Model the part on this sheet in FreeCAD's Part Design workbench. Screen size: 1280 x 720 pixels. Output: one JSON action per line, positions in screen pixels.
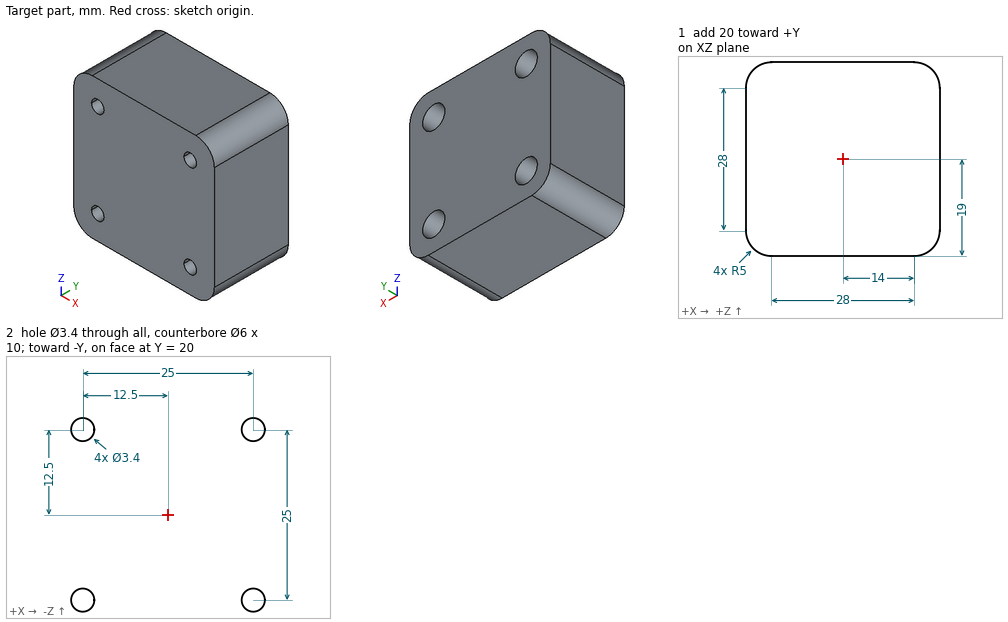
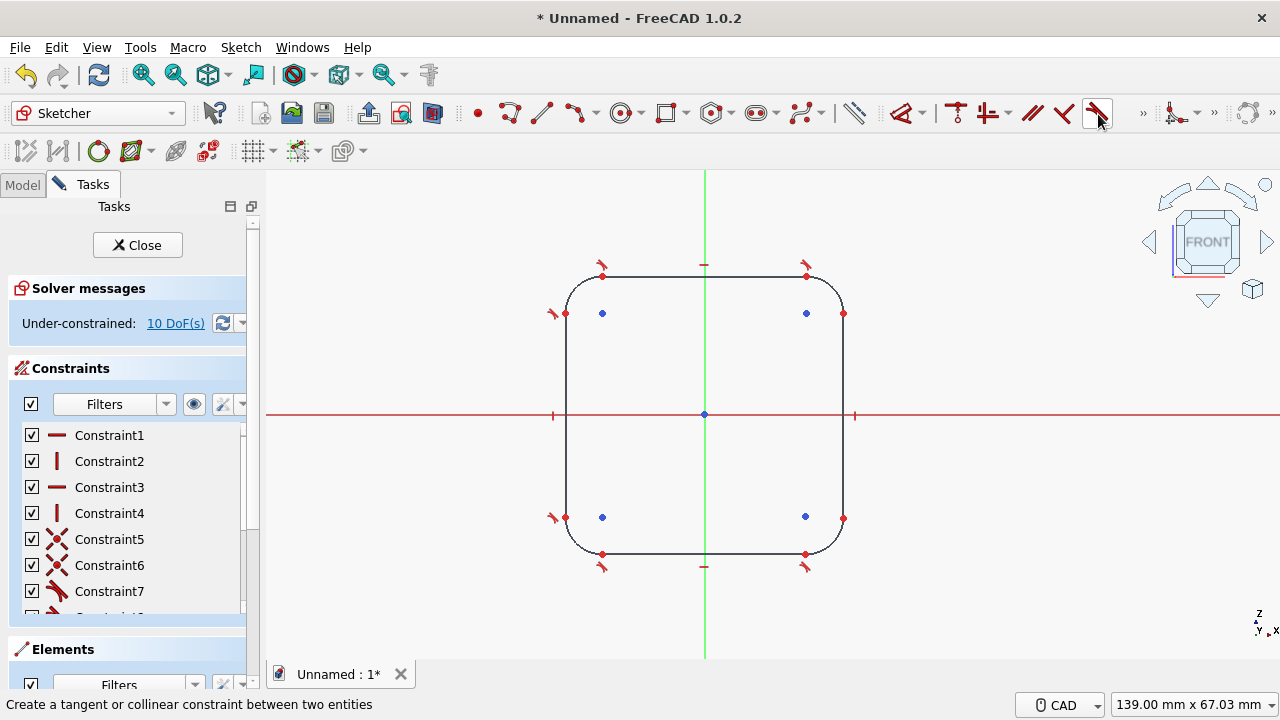
{"action": "left_click", "coordinate": [843, 375]}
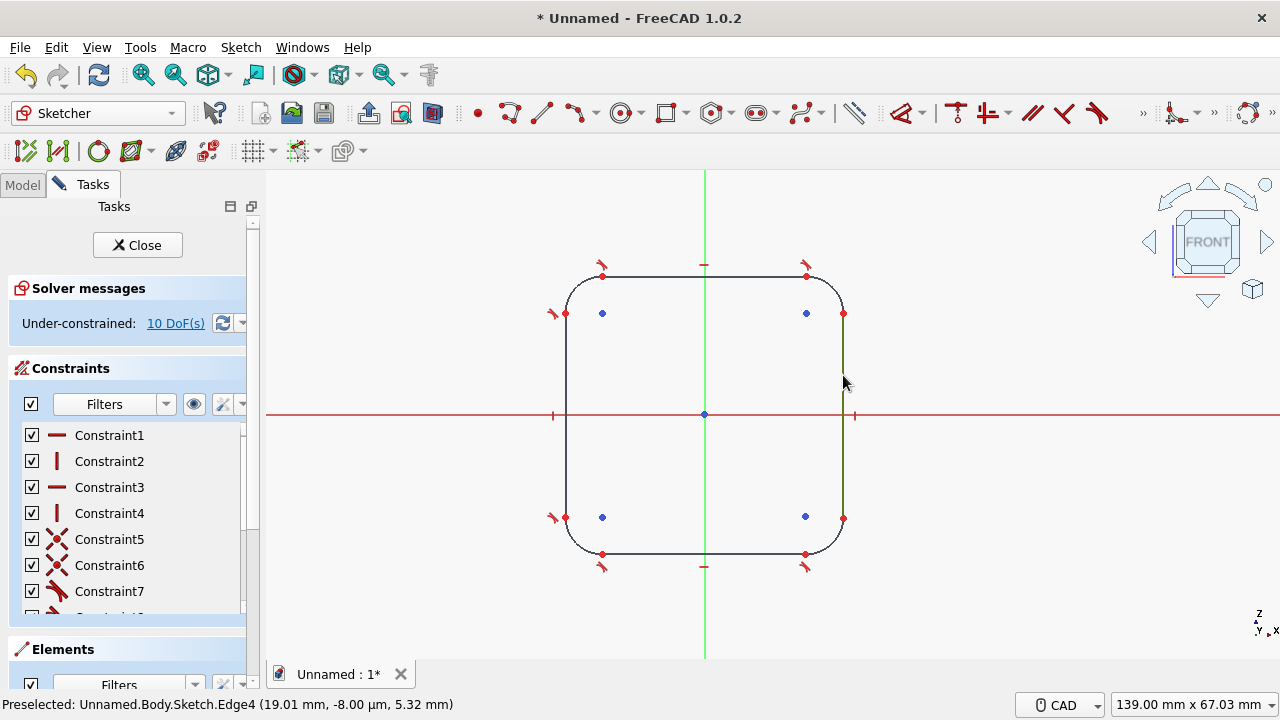
{"action": "left_click", "coordinate": [839, 297]}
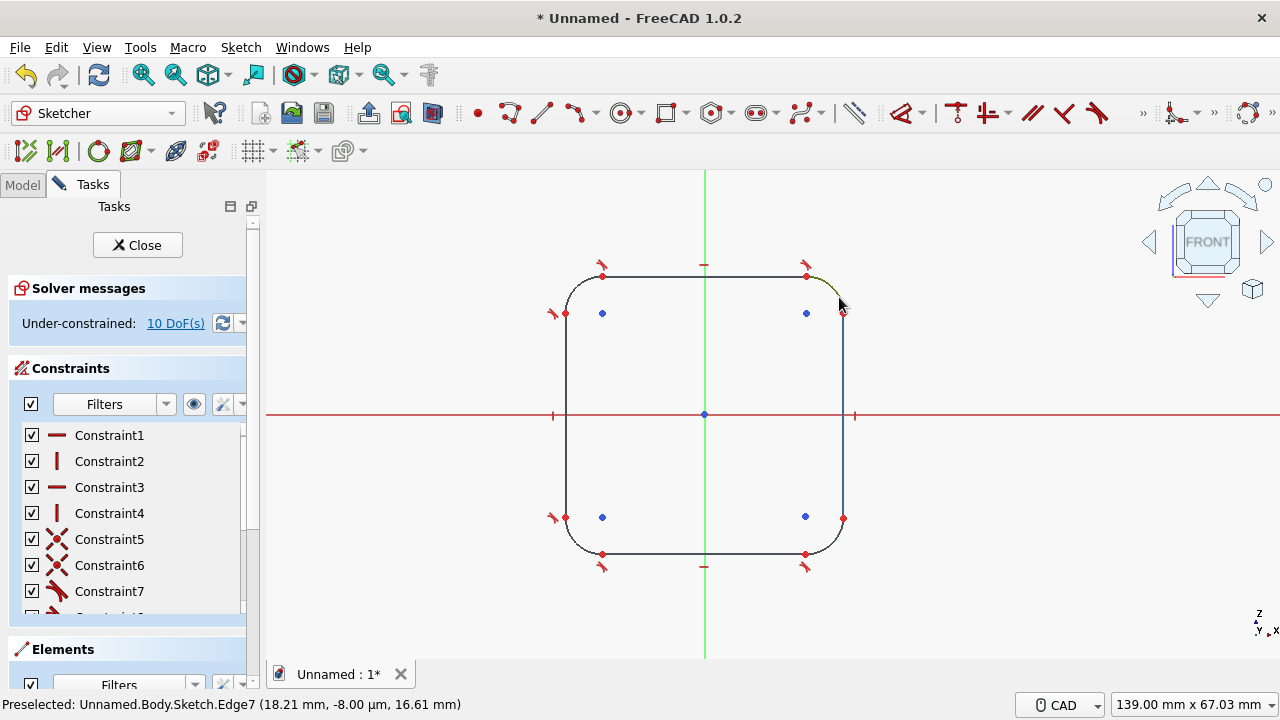
{"action": "left_click", "coordinate": [1098, 114]}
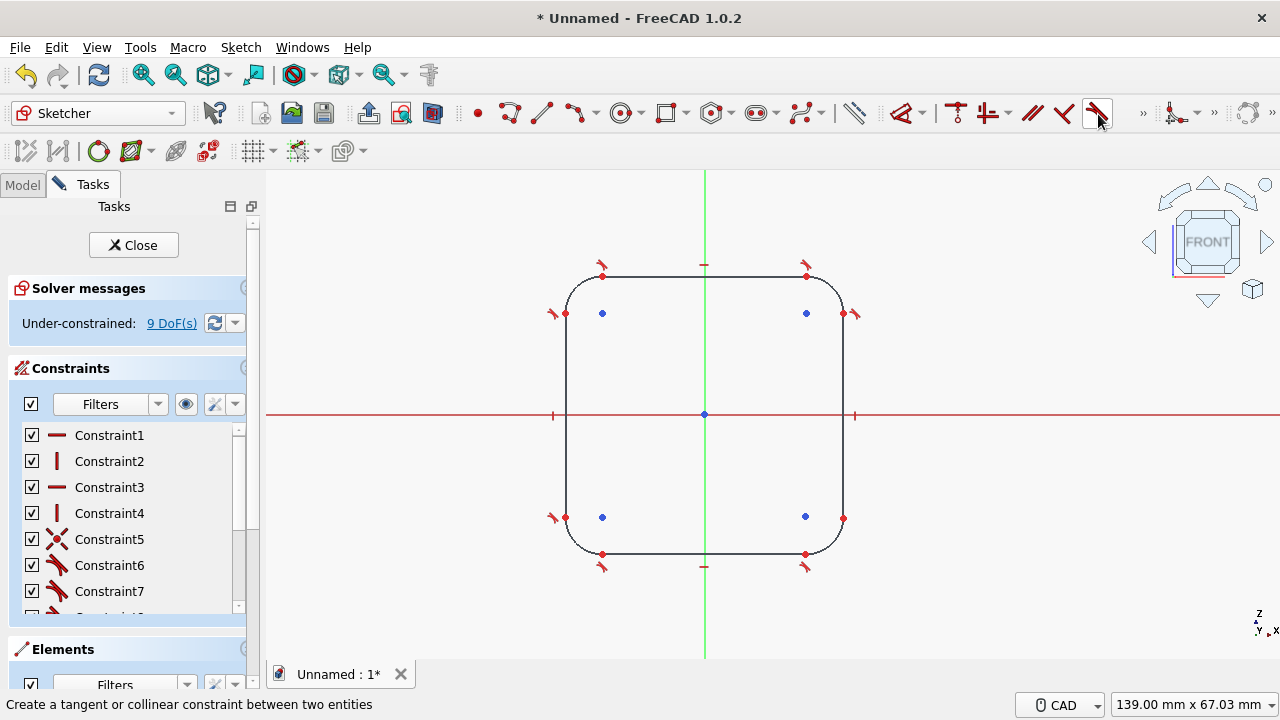
{"action": "left_click", "coordinate": [843, 375]}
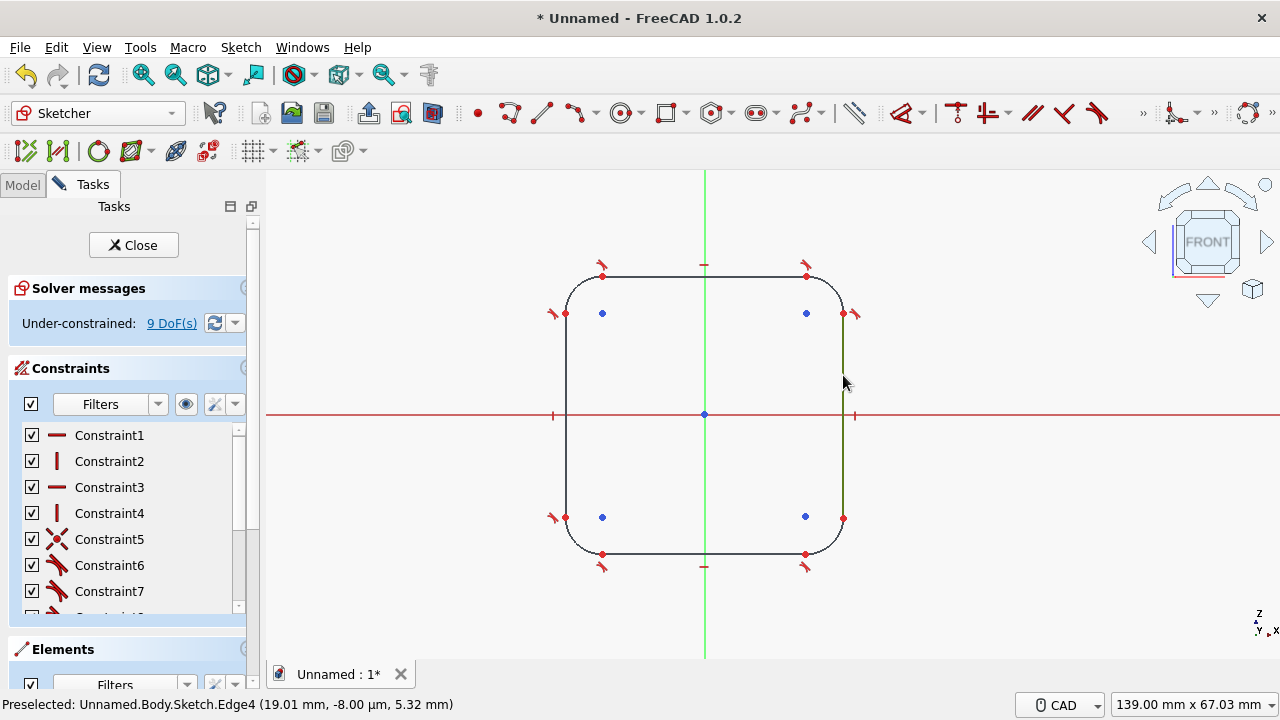
{"action": "left_click", "coordinate": [823, 550]}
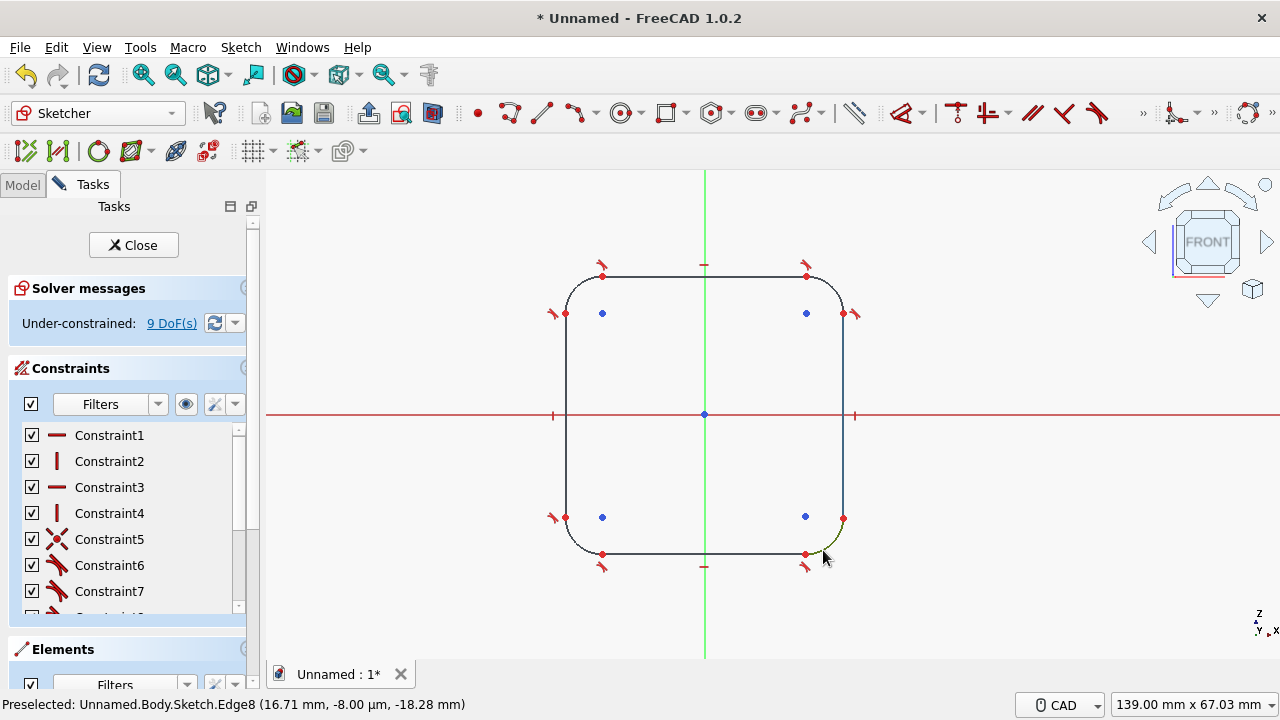
{"action": "left_click", "coordinate": [1098, 114]}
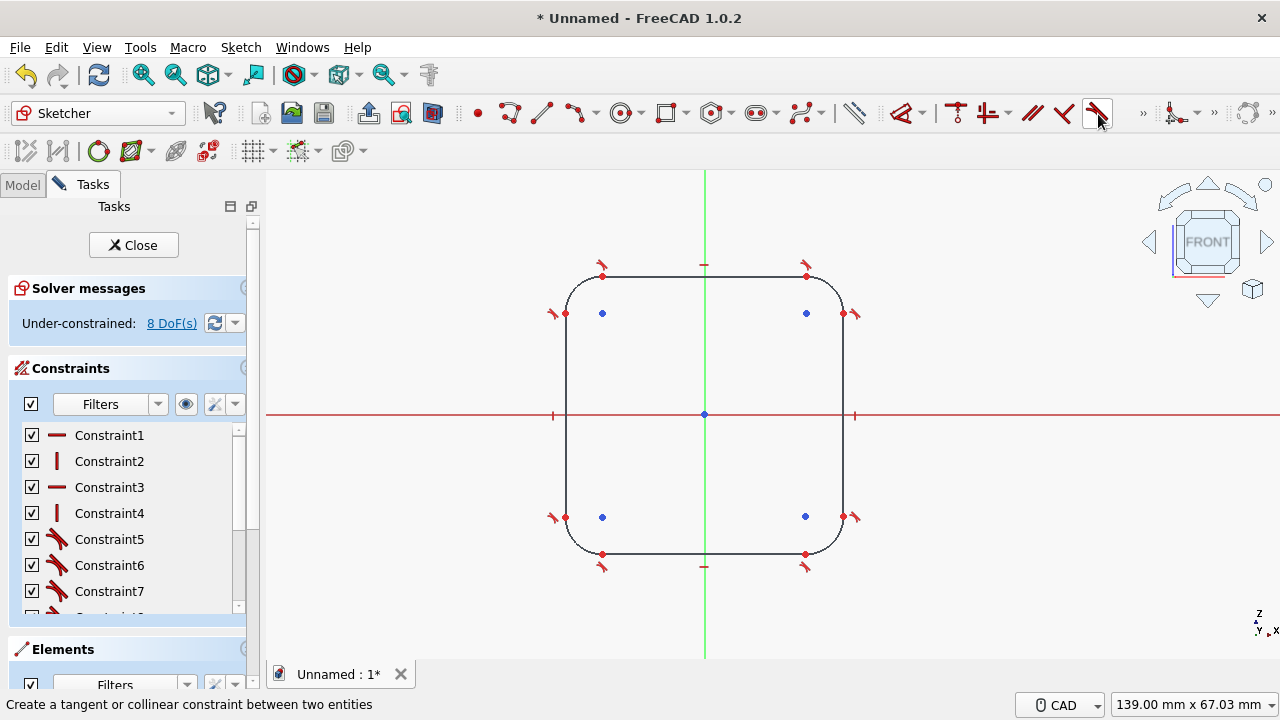
{"action": "left_click", "coordinate": [570, 534]}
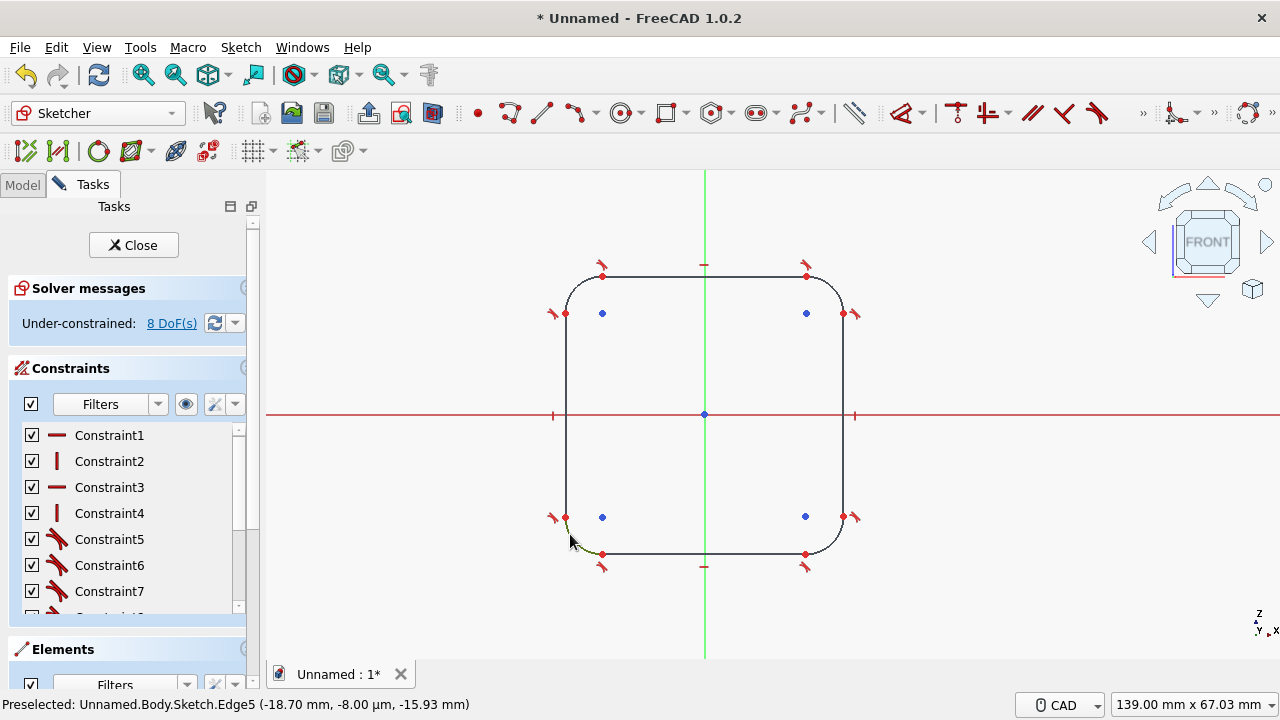
{"action": "left_click", "coordinate": [586, 281]}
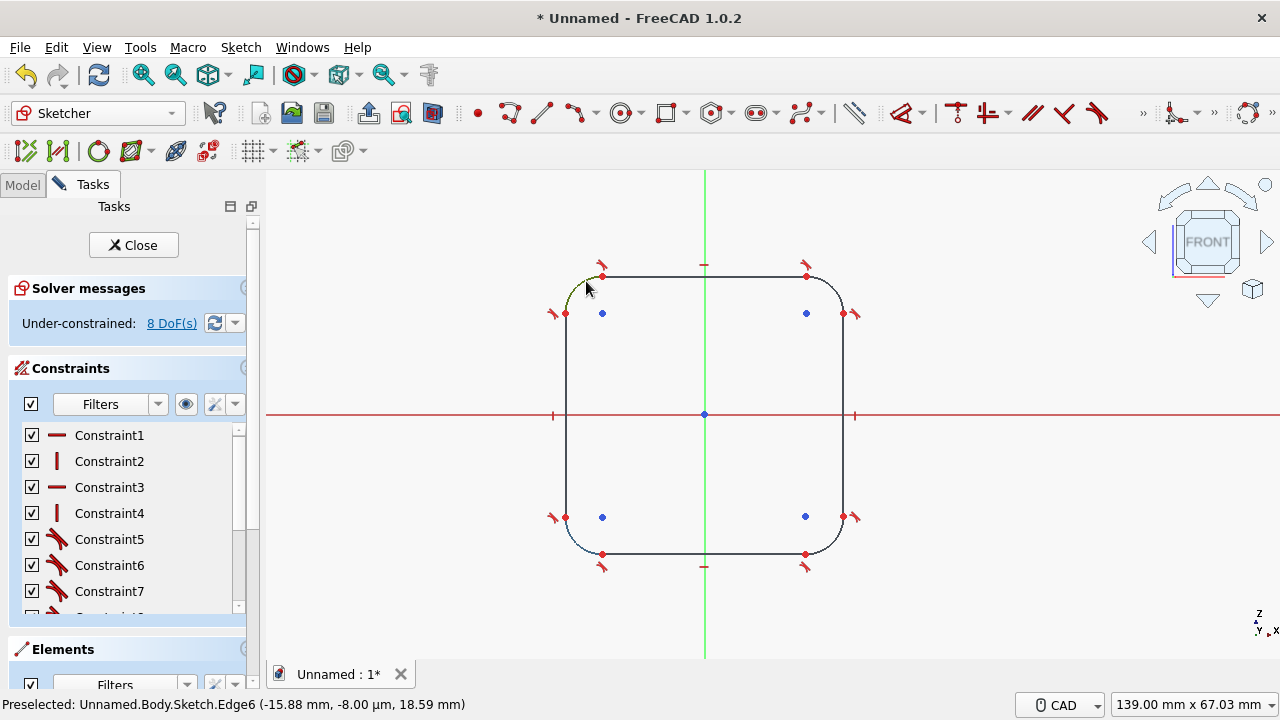
{"action": "left_click", "coordinate": [839, 297]}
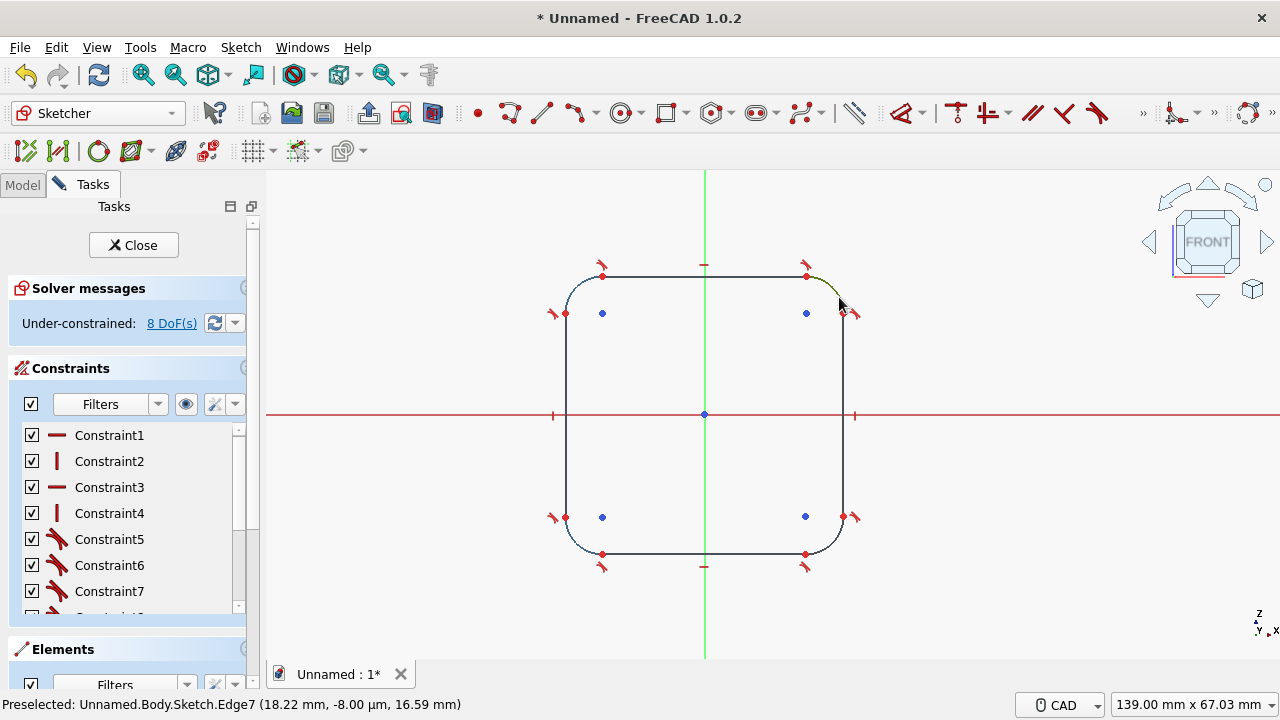
{"action": "left_click", "coordinate": [823, 550]}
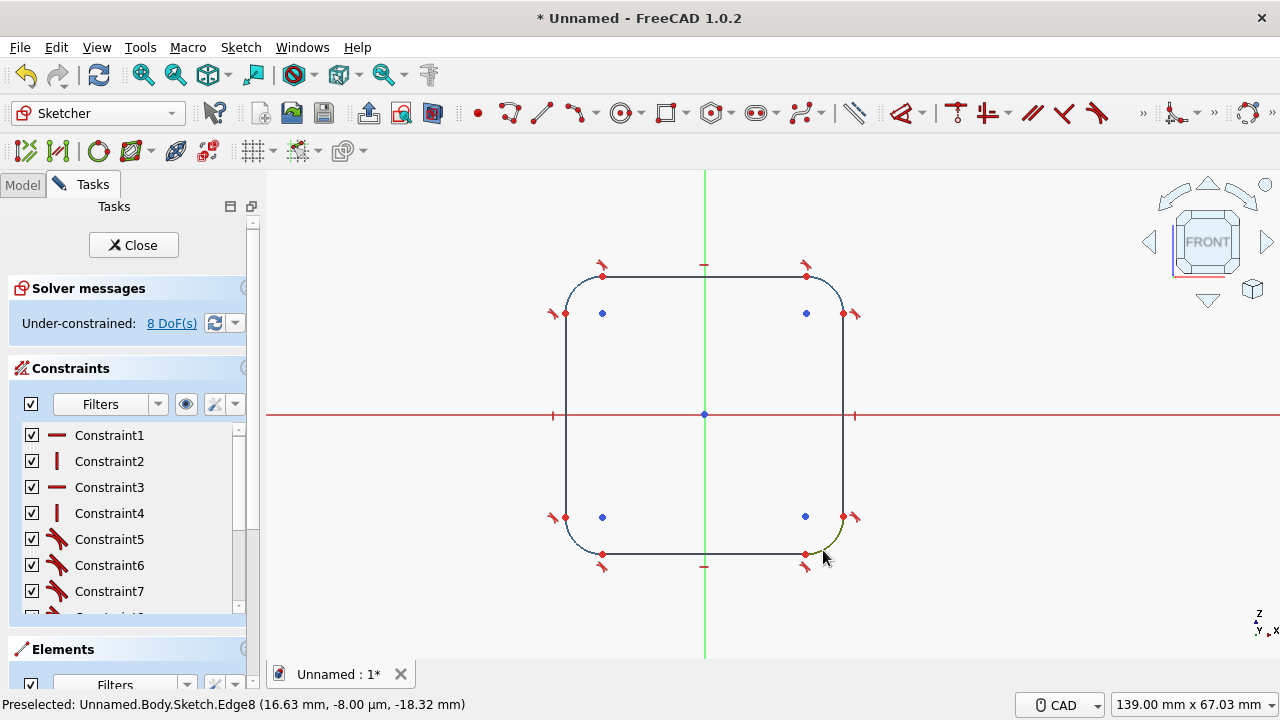
{"action": "key", "text": "e"}